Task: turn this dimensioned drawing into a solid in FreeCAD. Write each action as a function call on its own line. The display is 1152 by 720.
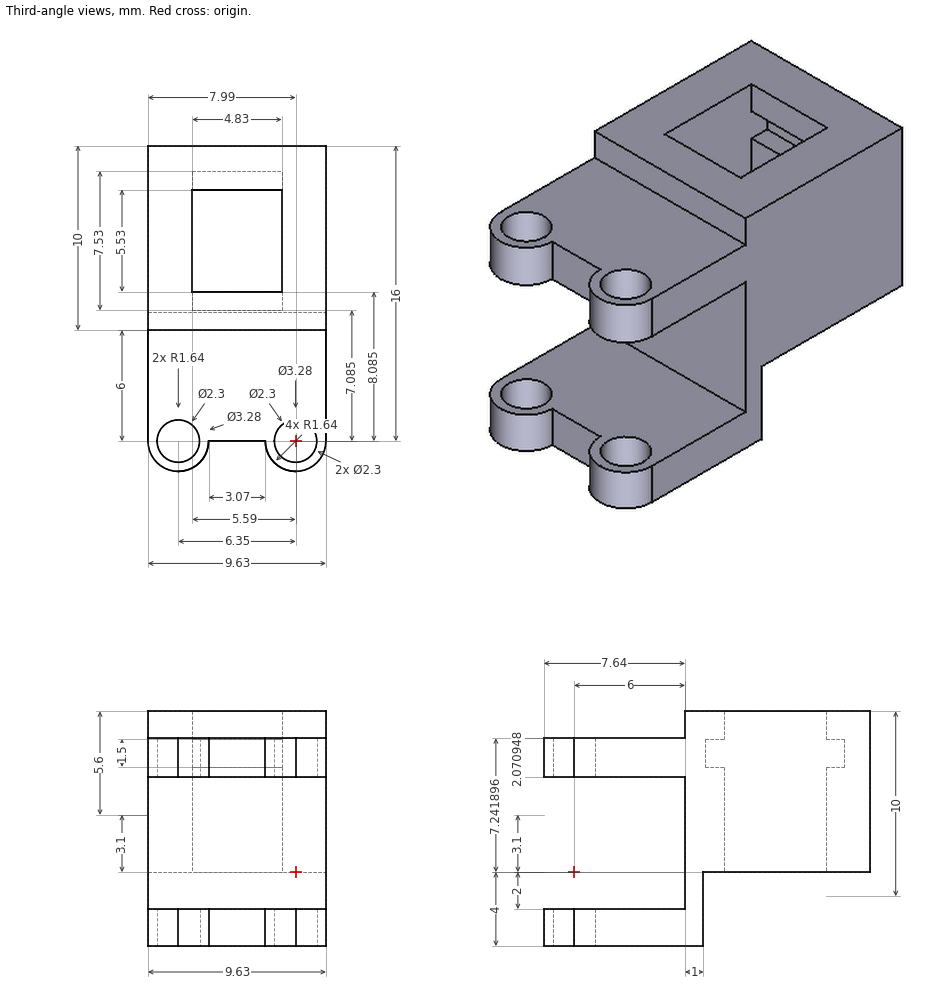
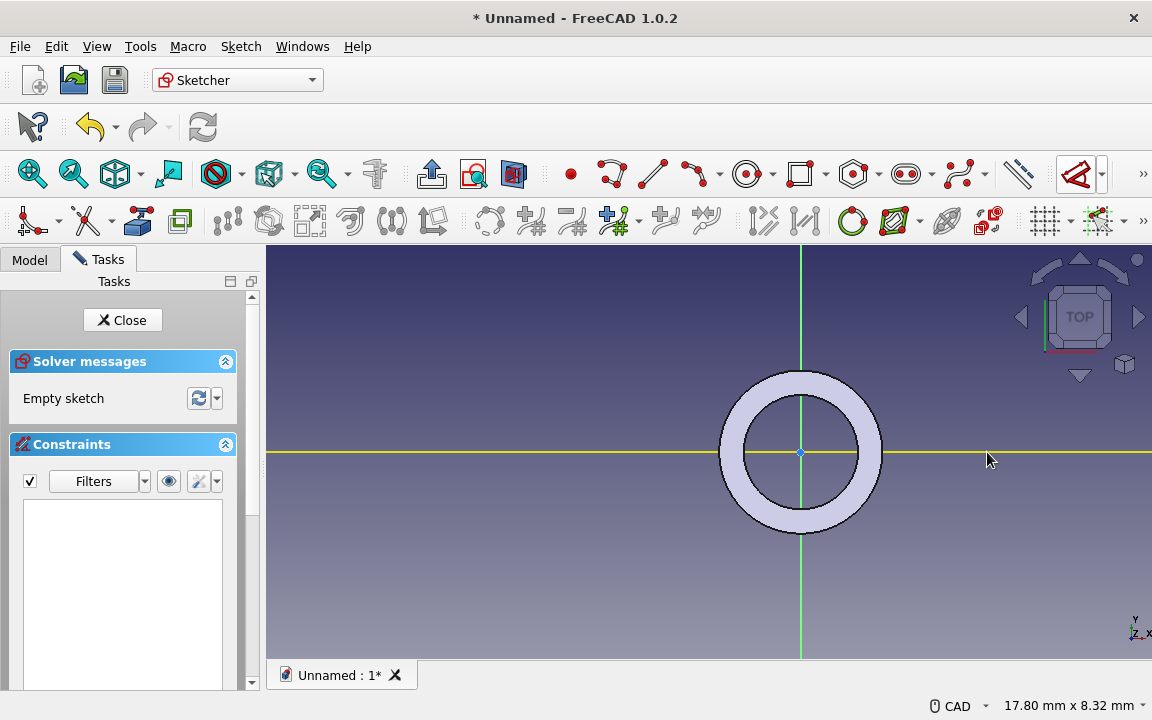
key(g)
key(c)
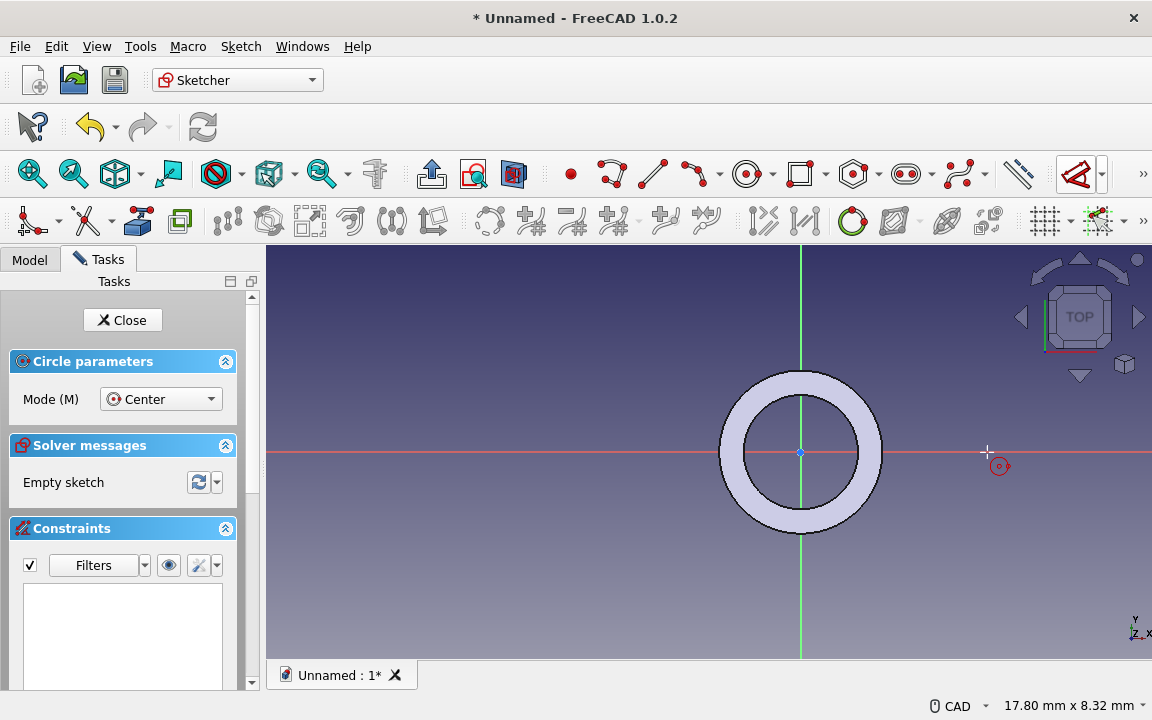
click(485, 452)
click(543, 394)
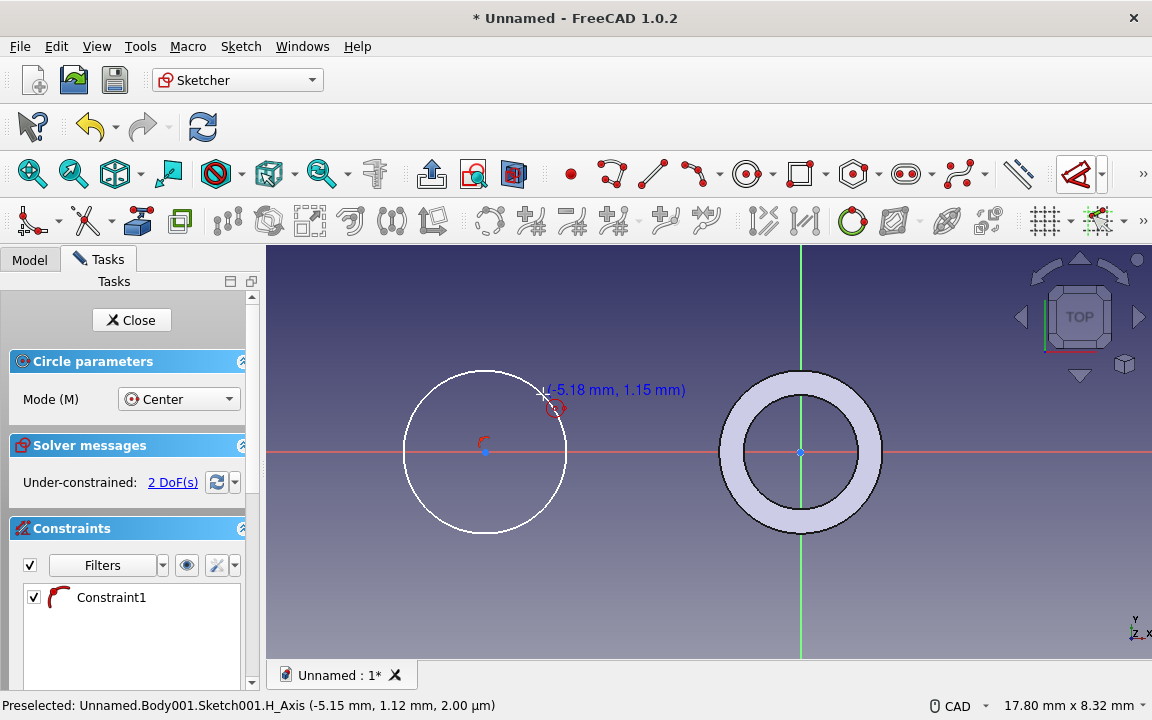
click(485, 452)
click(525, 412)
key(Escape)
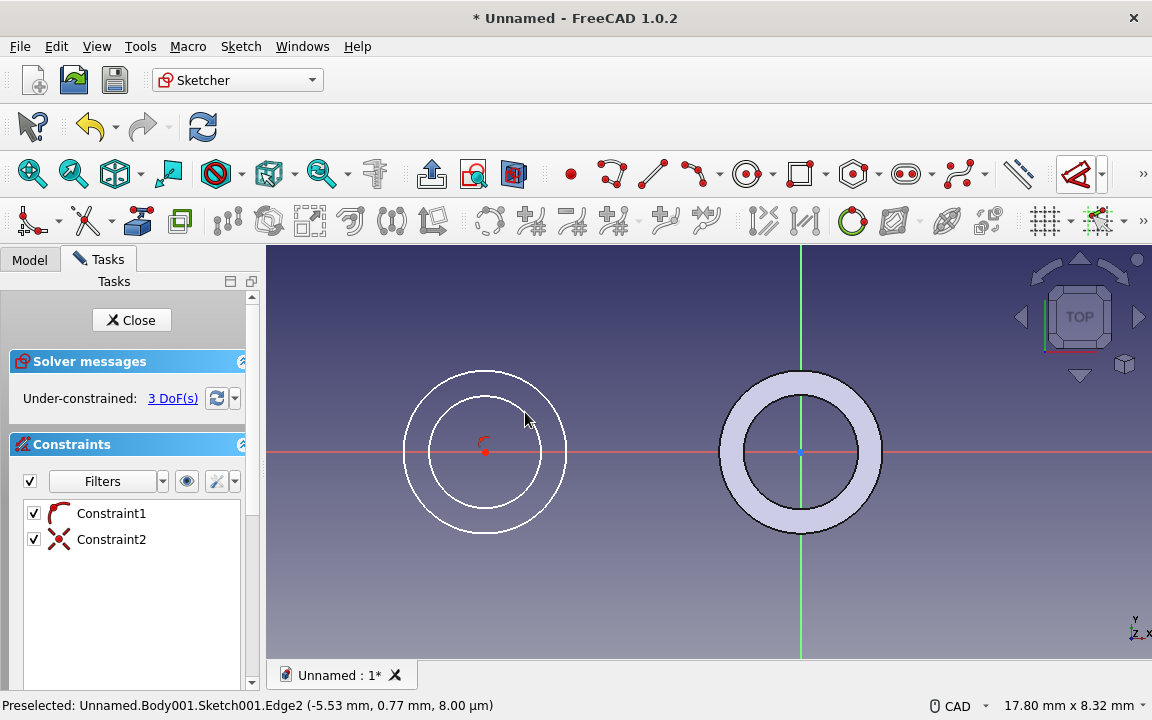
click(1076, 174)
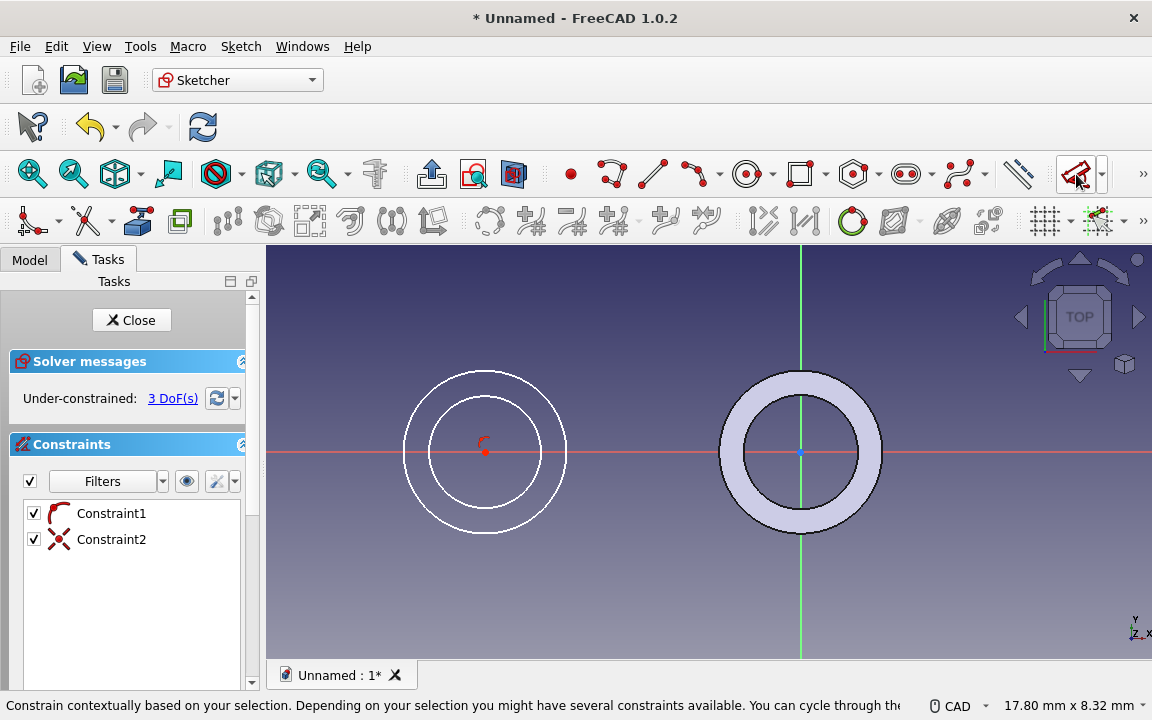
click(542, 394)
click(564, 371)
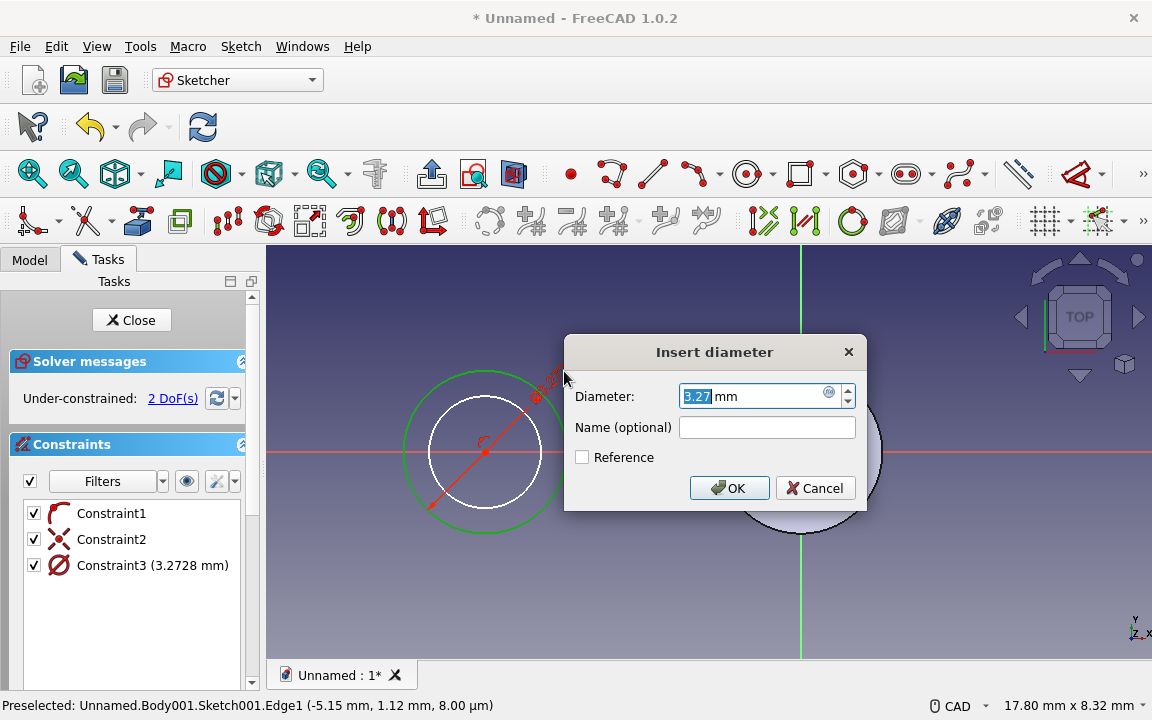
text(3.28)
key(Return)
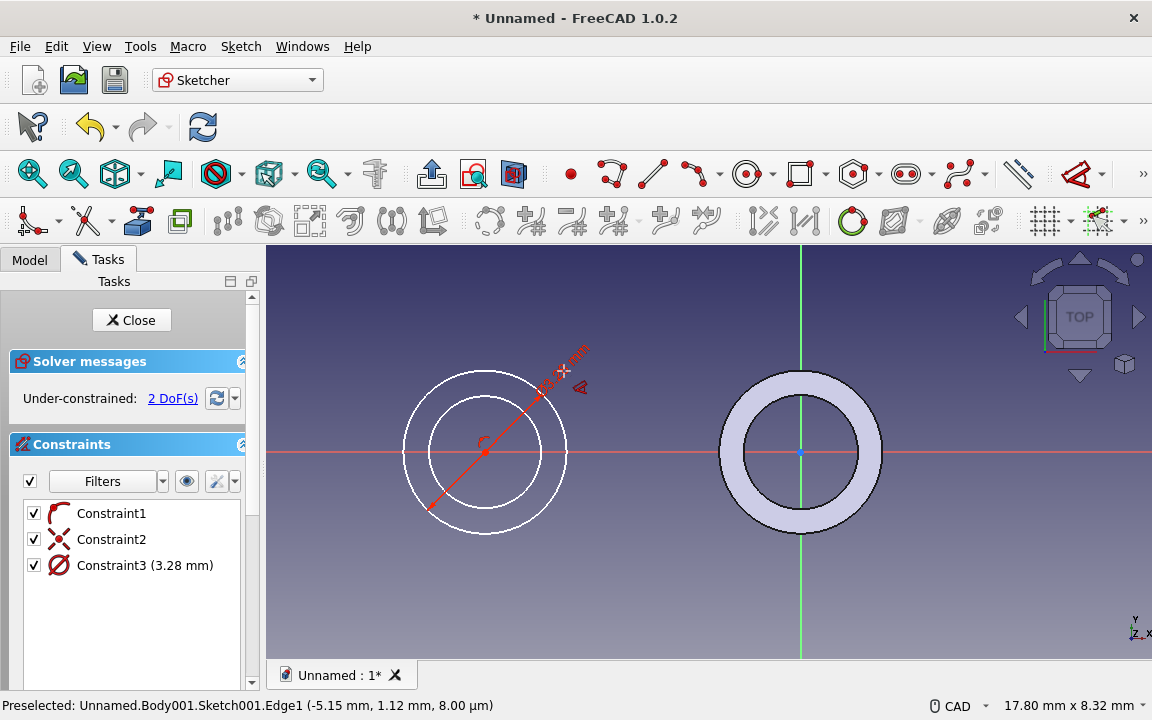
click(524, 412)
click(591, 419)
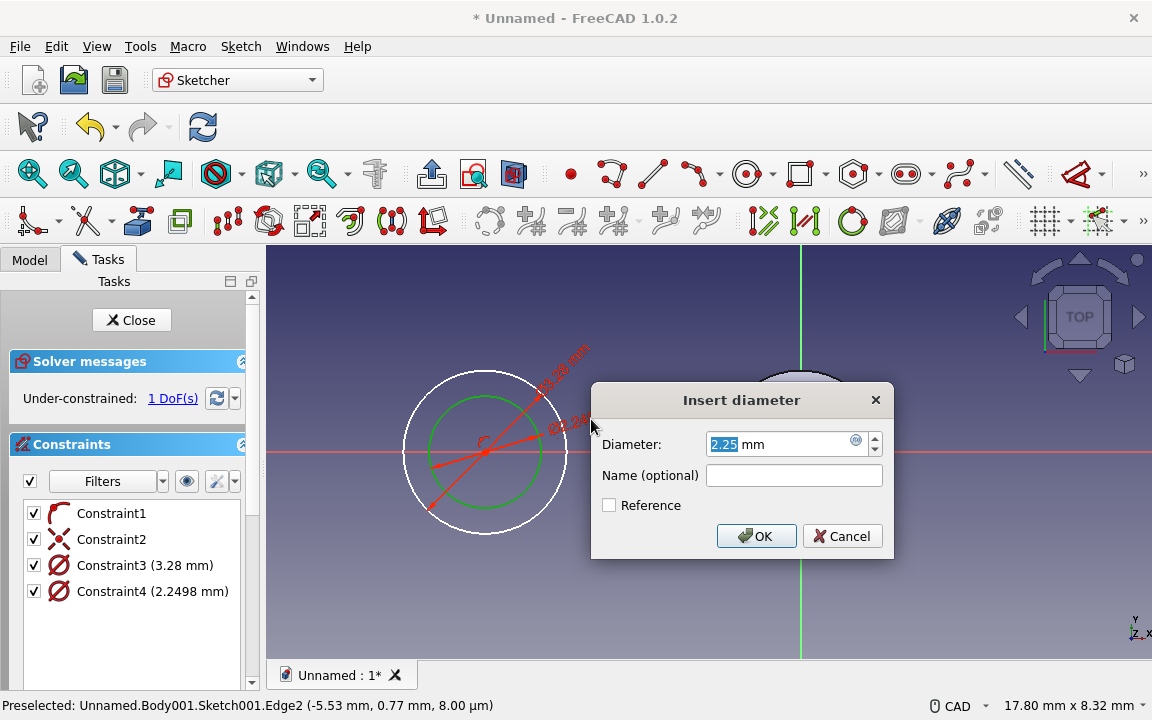
text(2.3)
key(Return)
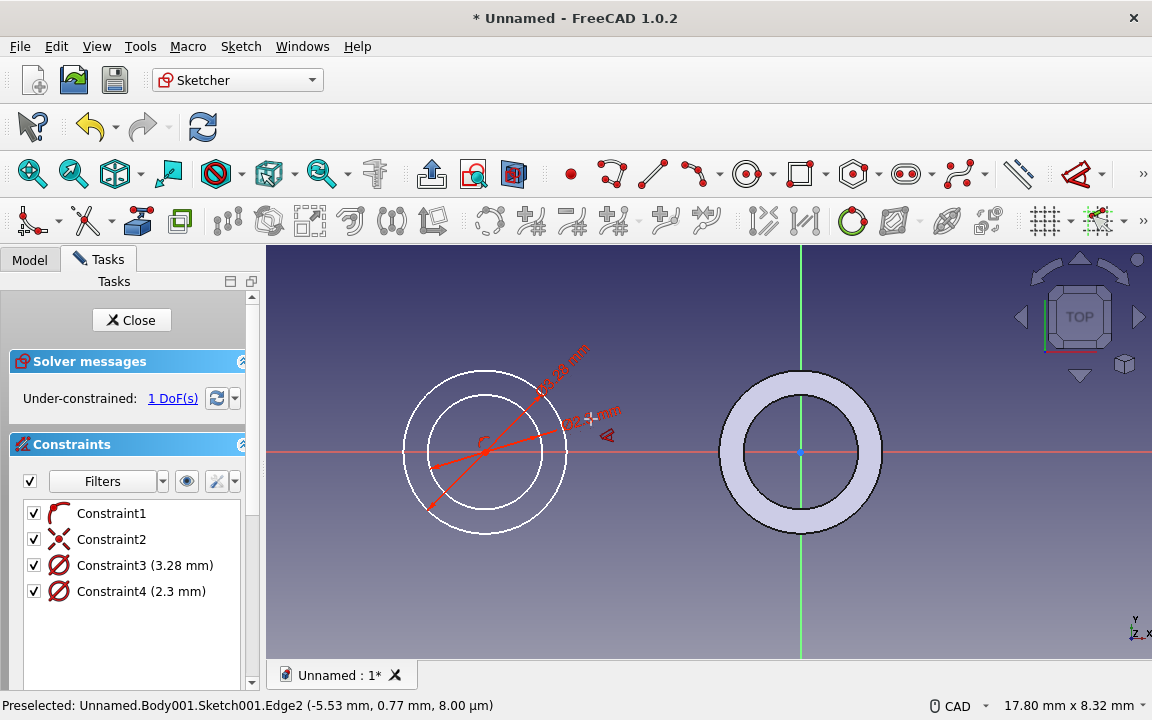
click(485, 452)
click(643, 486)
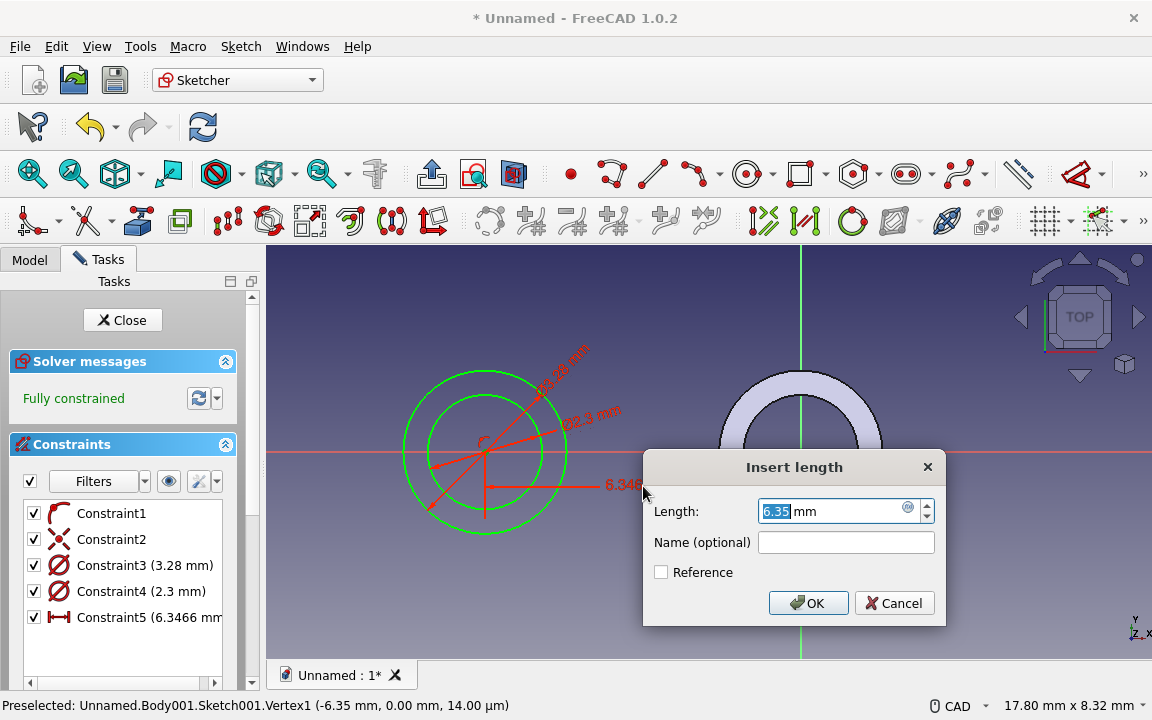
text(6.35)
key(Return)
key(Escape)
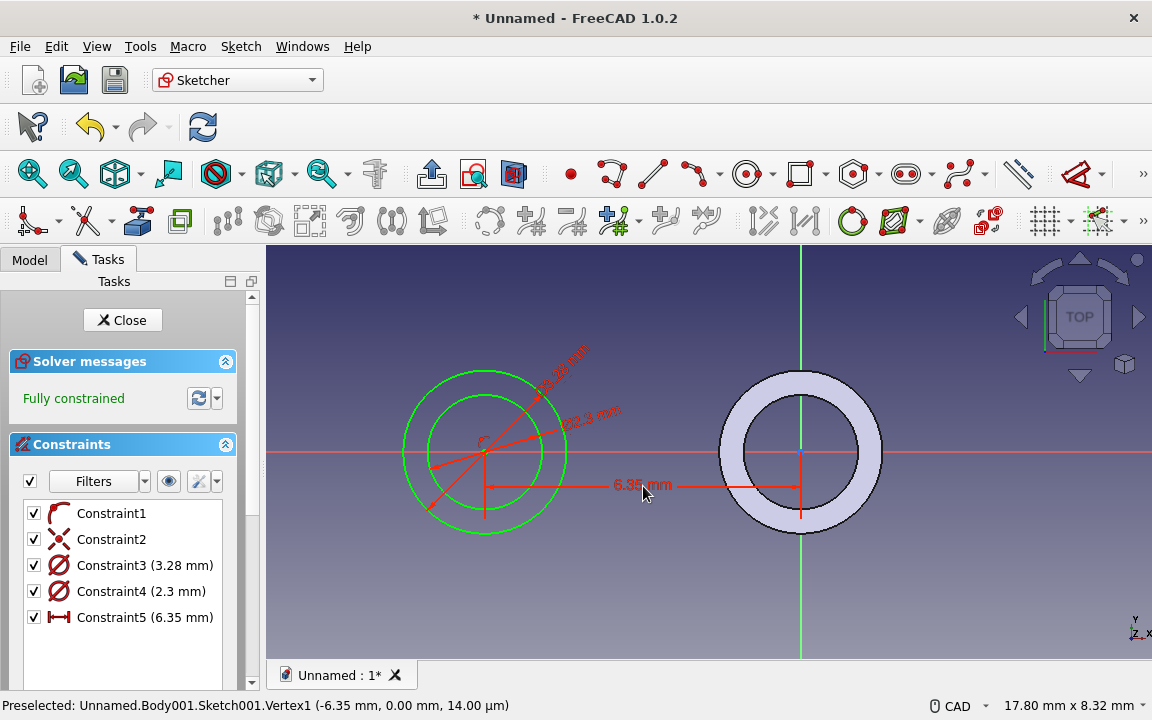
click(123, 320)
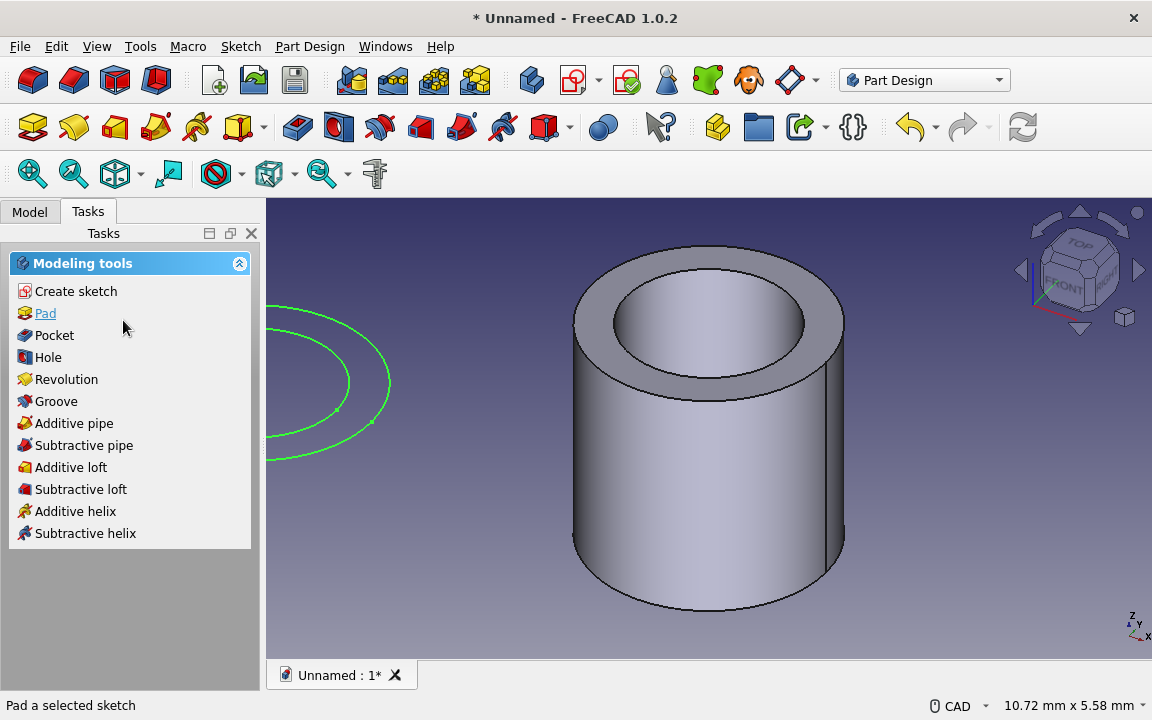
click(33, 128)